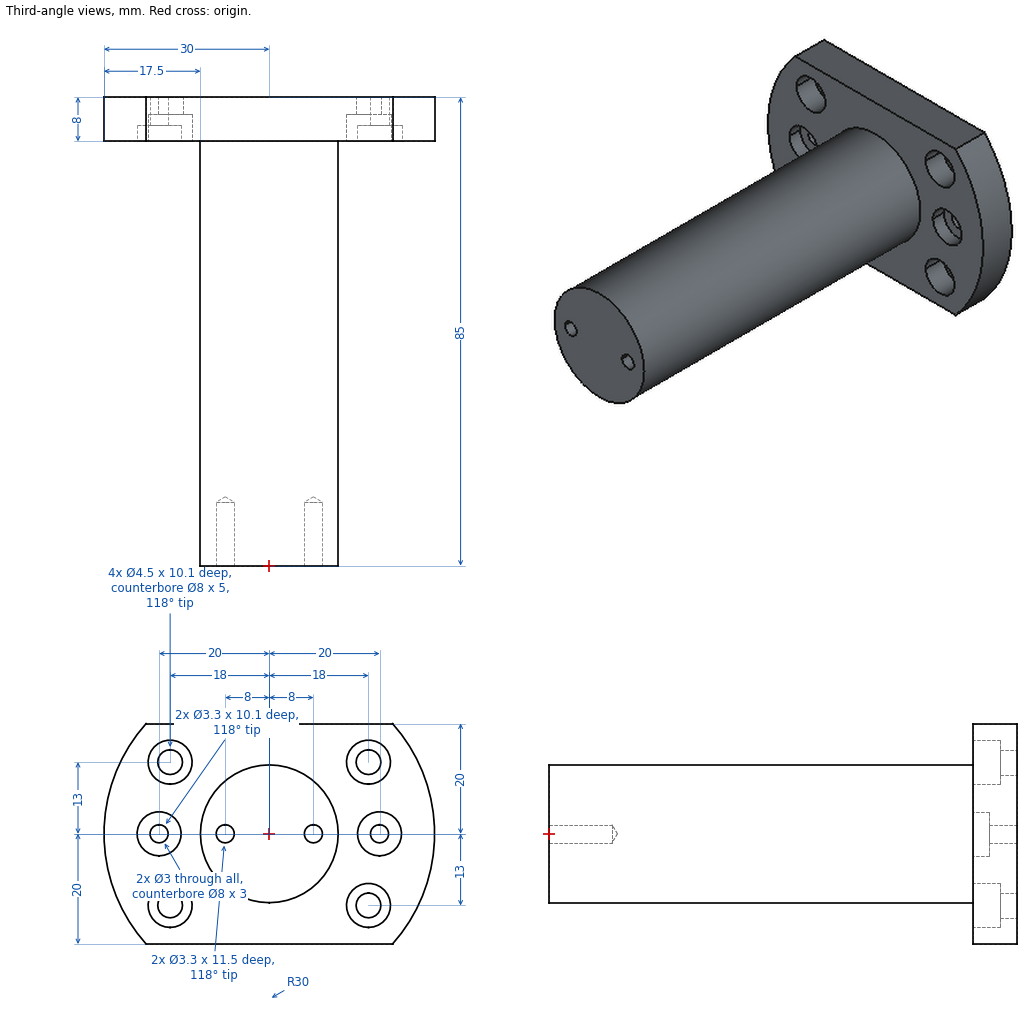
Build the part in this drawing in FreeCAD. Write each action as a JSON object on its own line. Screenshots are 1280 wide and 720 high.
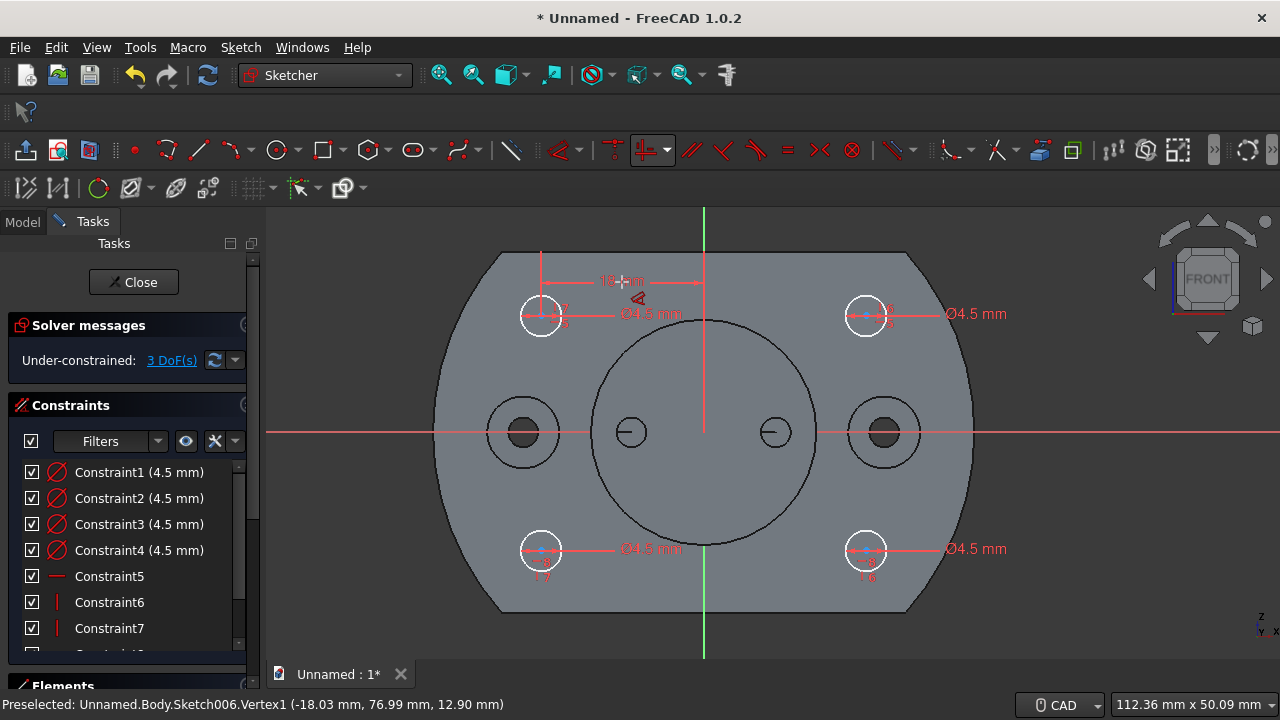
{"action": "left_click", "coordinate": [541, 316]}
{"action": "left_click", "coordinate": [507, 374]}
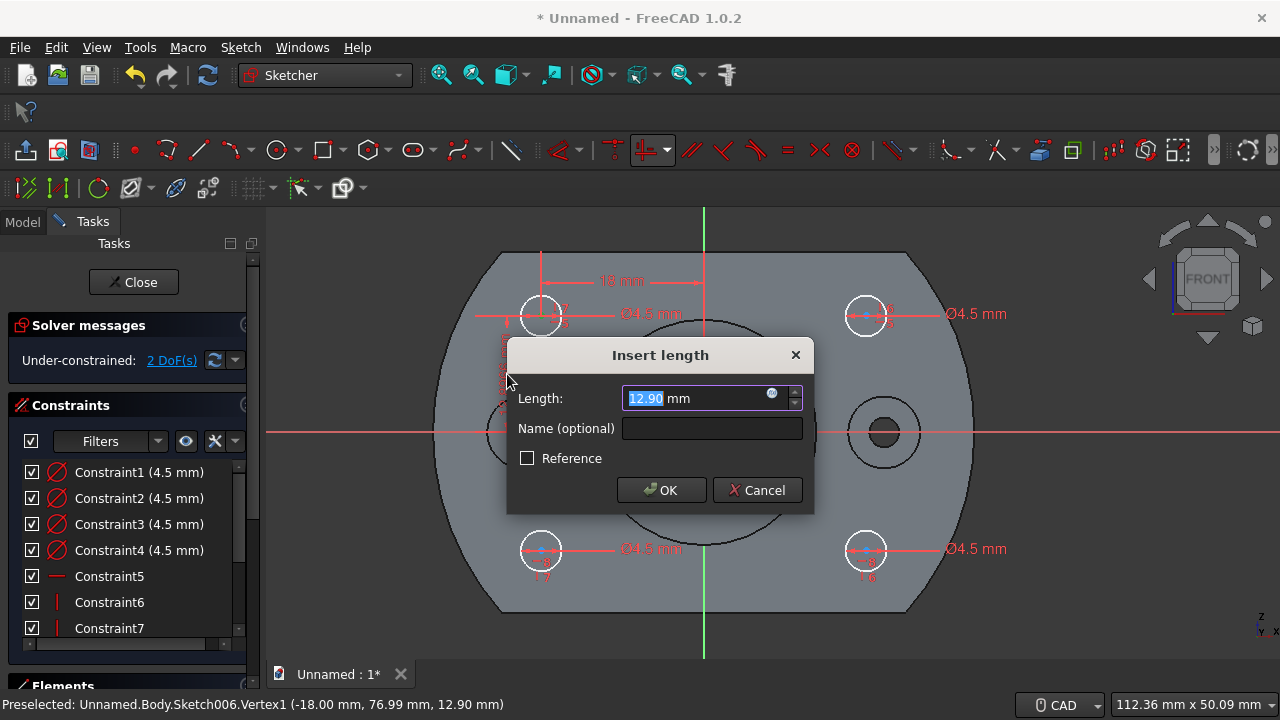
{"action": "type", "text": "13"}
{"action": "key", "text": "Return"}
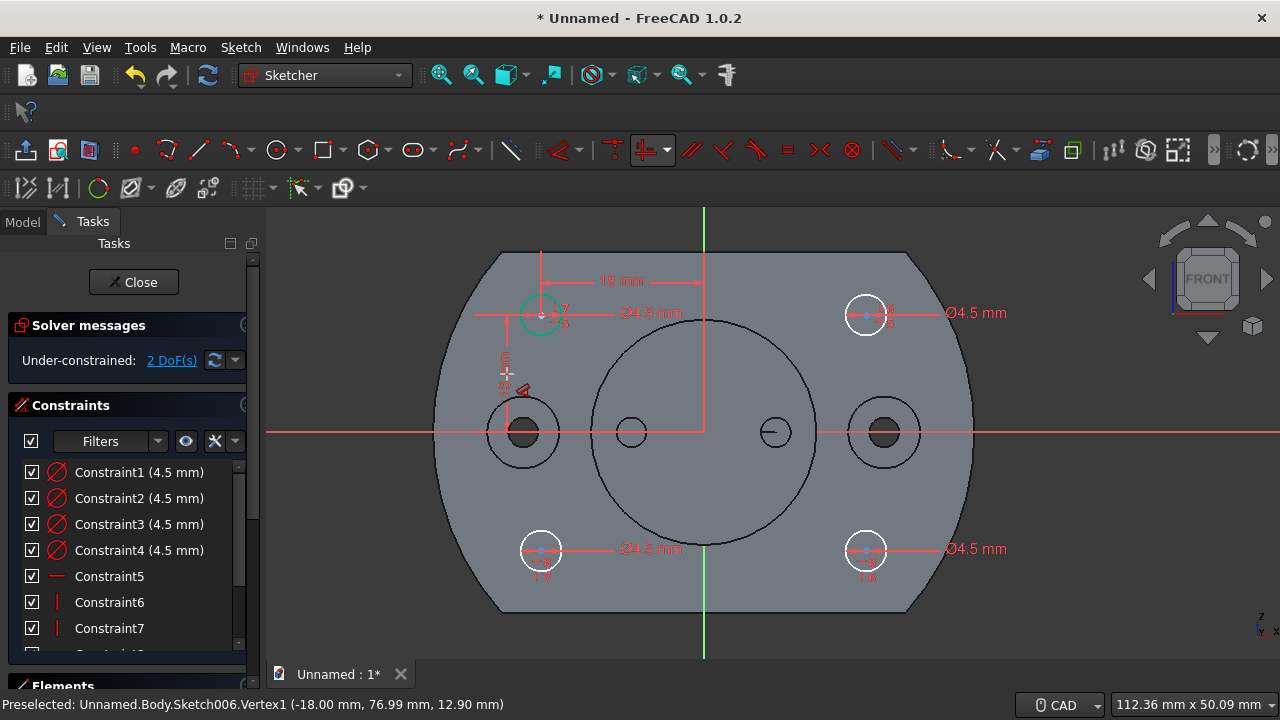
{"action": "left_click", "coordinate": [866, 315]}
{"action": "left_click", "coordinate": [785, 281]}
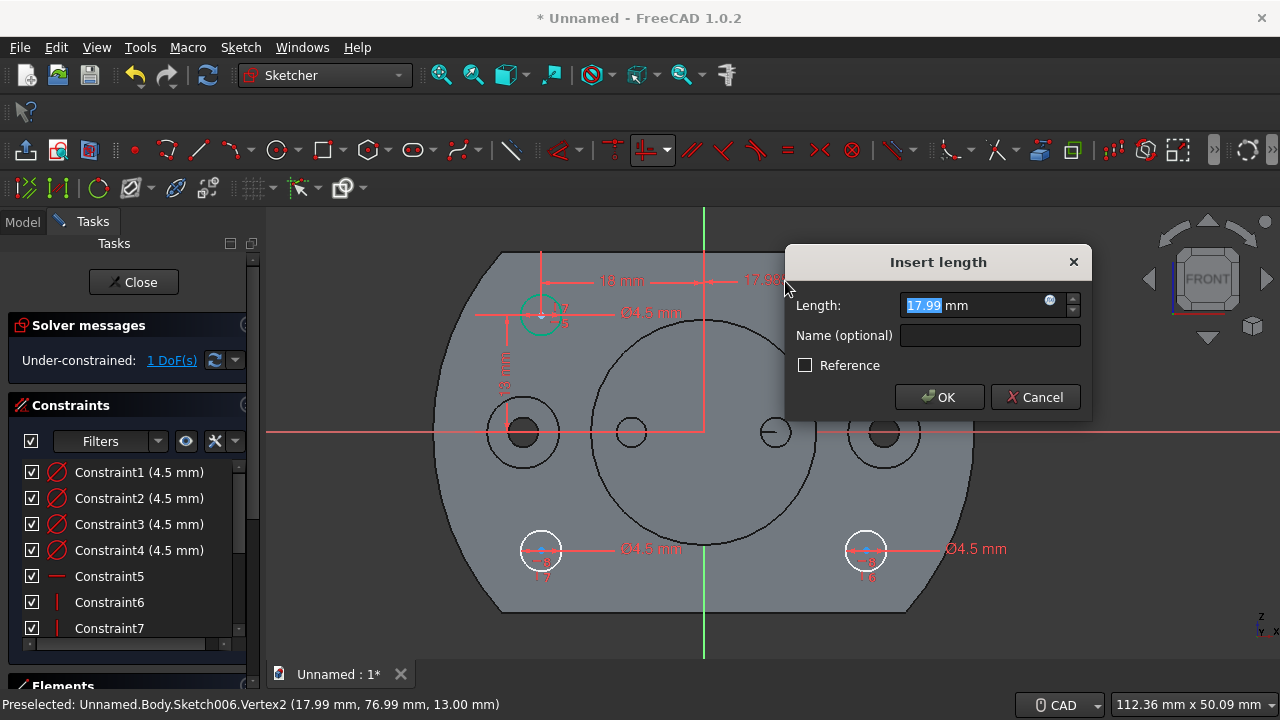
{"action": "type", "text": "18"}
{"action": "key", "text": "Return"}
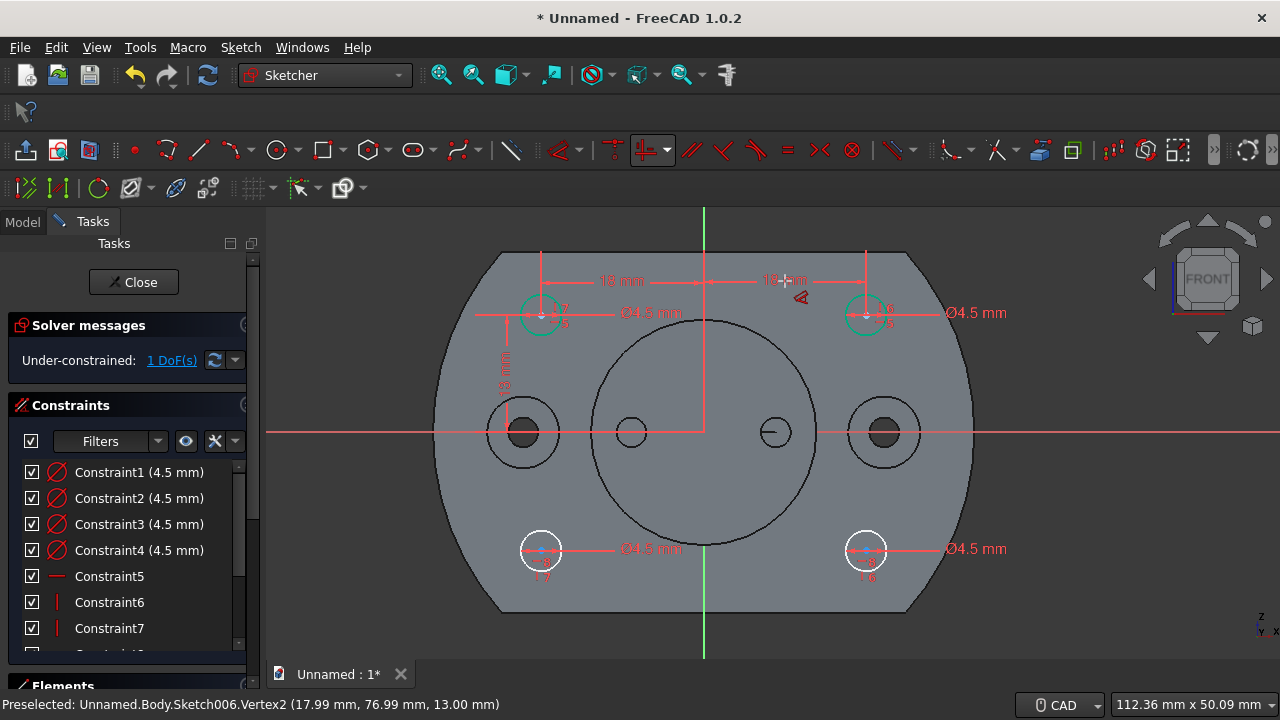
{"action": "left_click", "coordinate": [866, 551]}
{"action": "left_click", "coordinate": [900, 492]}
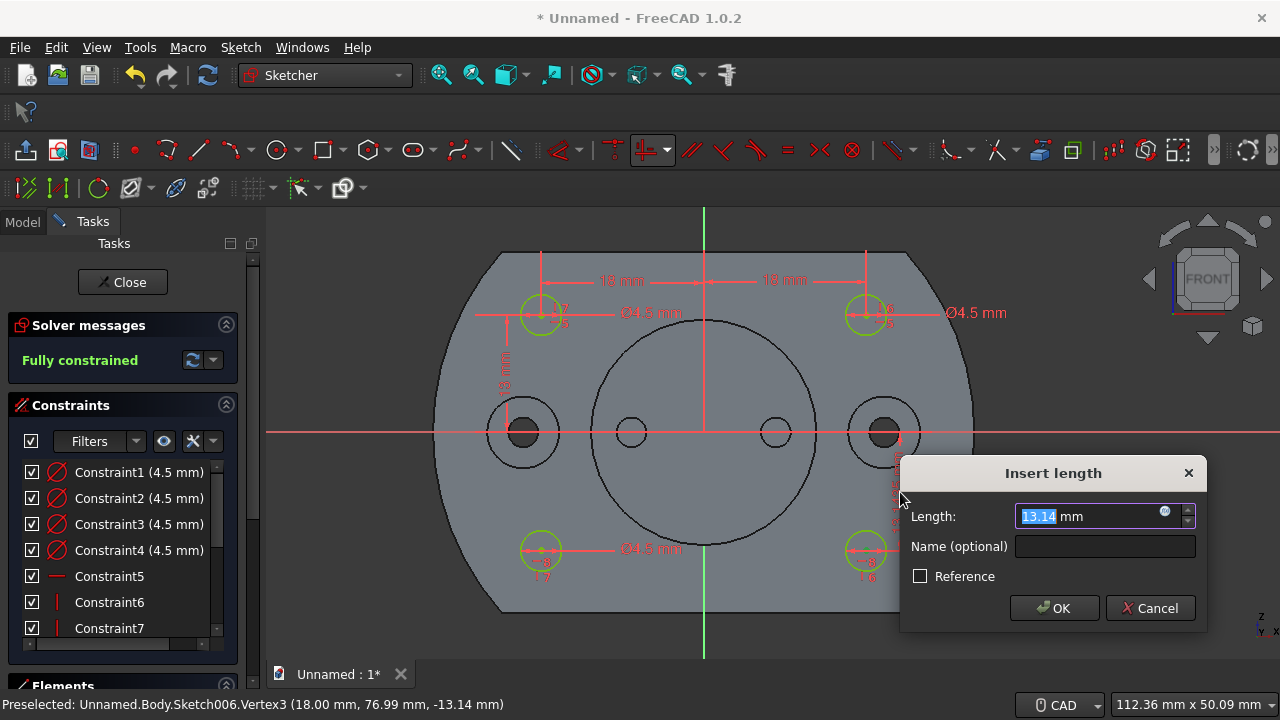
{"action": "type", "text": "13"}
{"action": "key", "text": "Return"}
{"action": "key", "text": "Escape"}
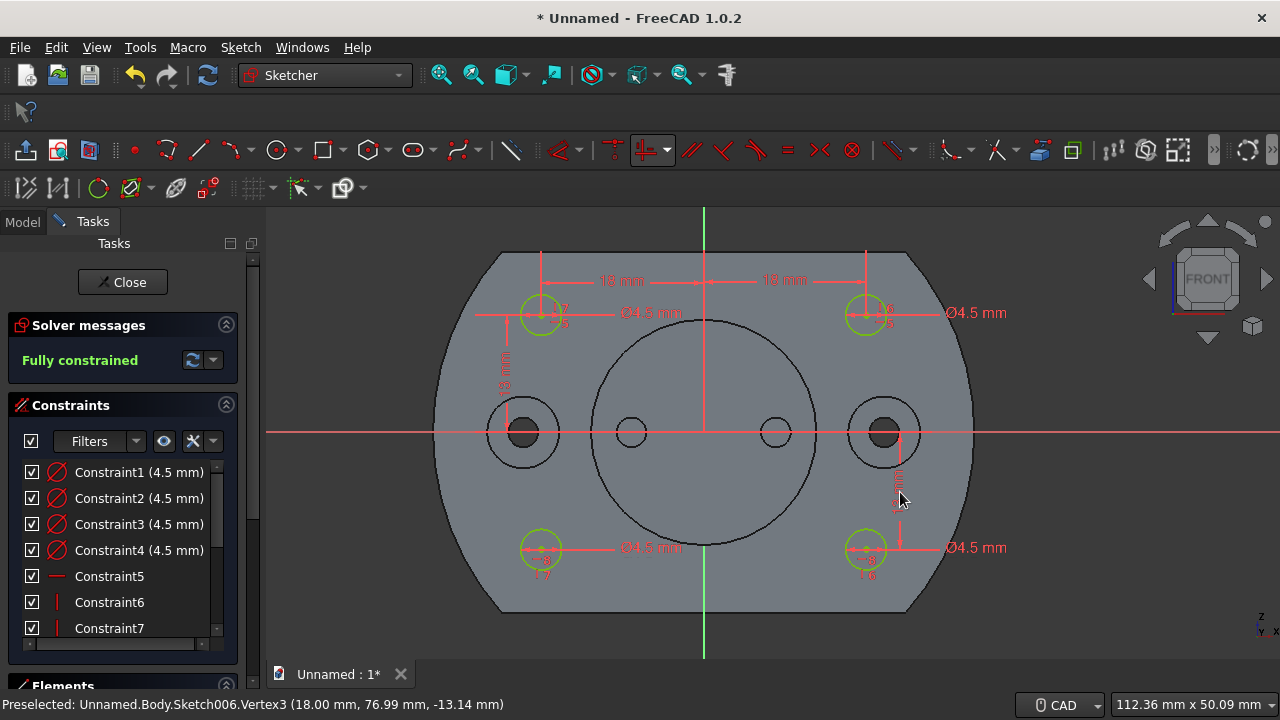
{"action": "left_click", "coordinate": [123, 282]}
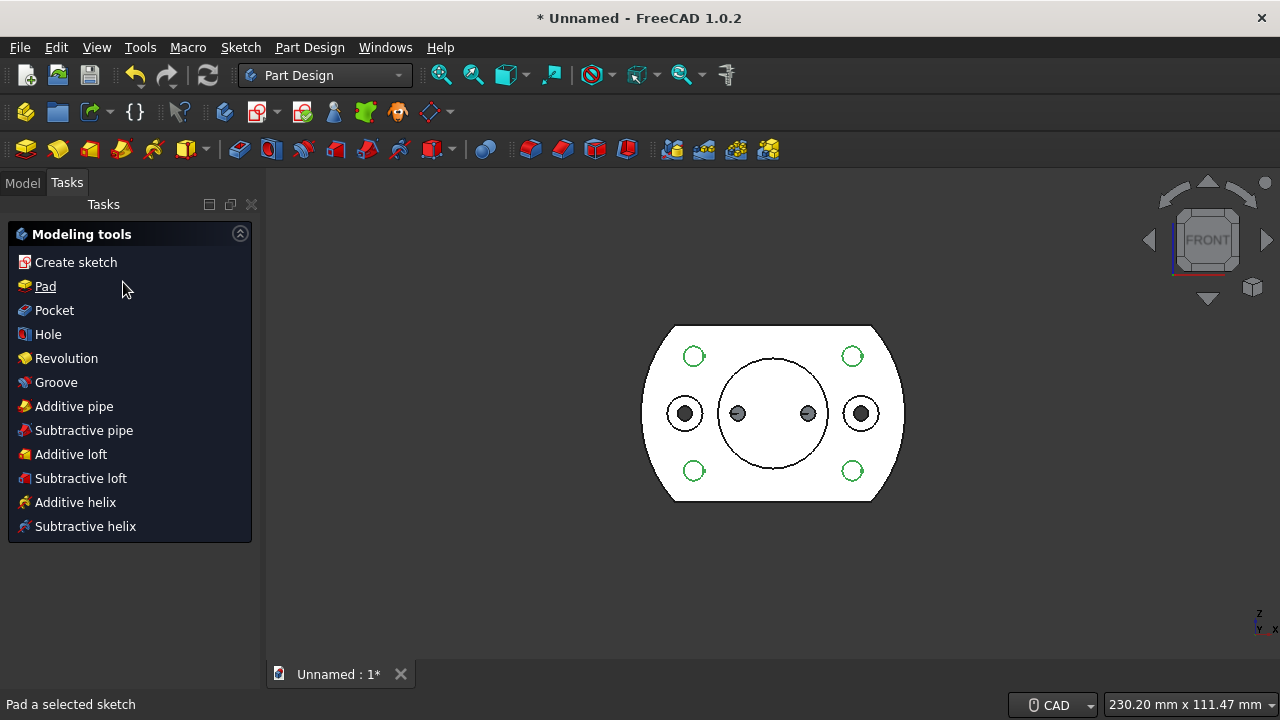
{"action": "left_click", "coordinate": [272, 150]}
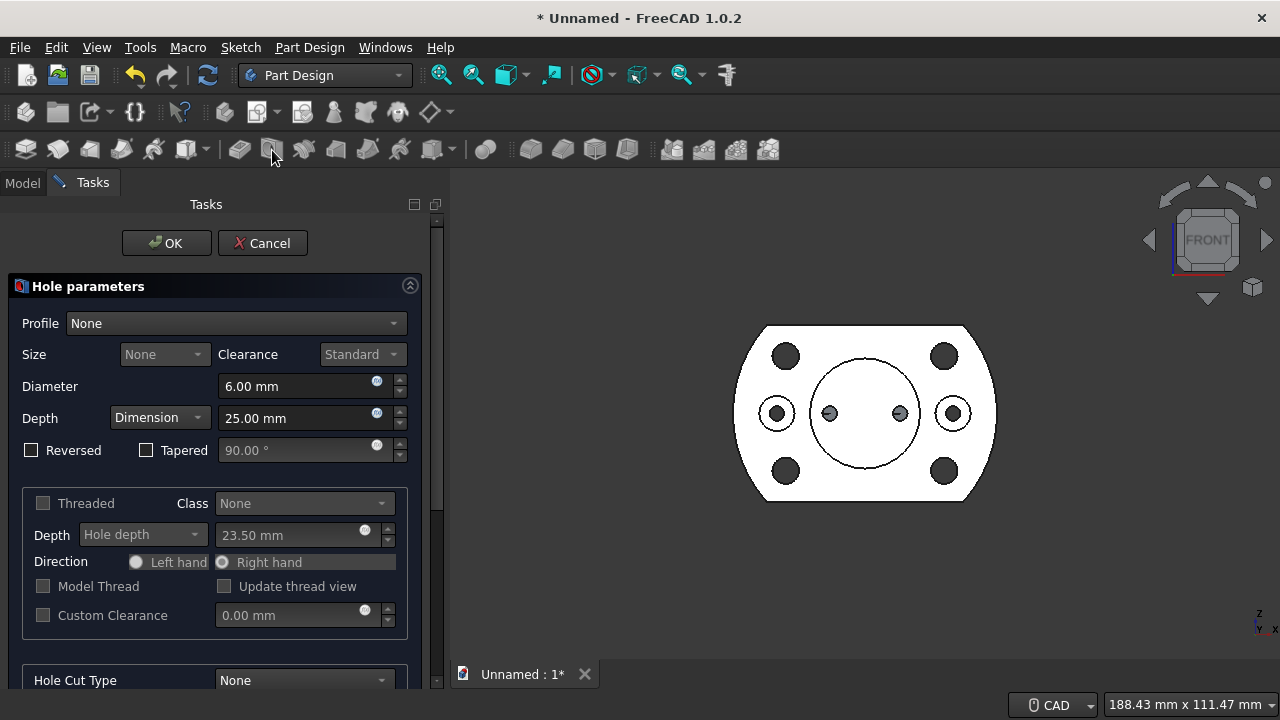
{"action": "triple_click", "coordinate": [305, 386]}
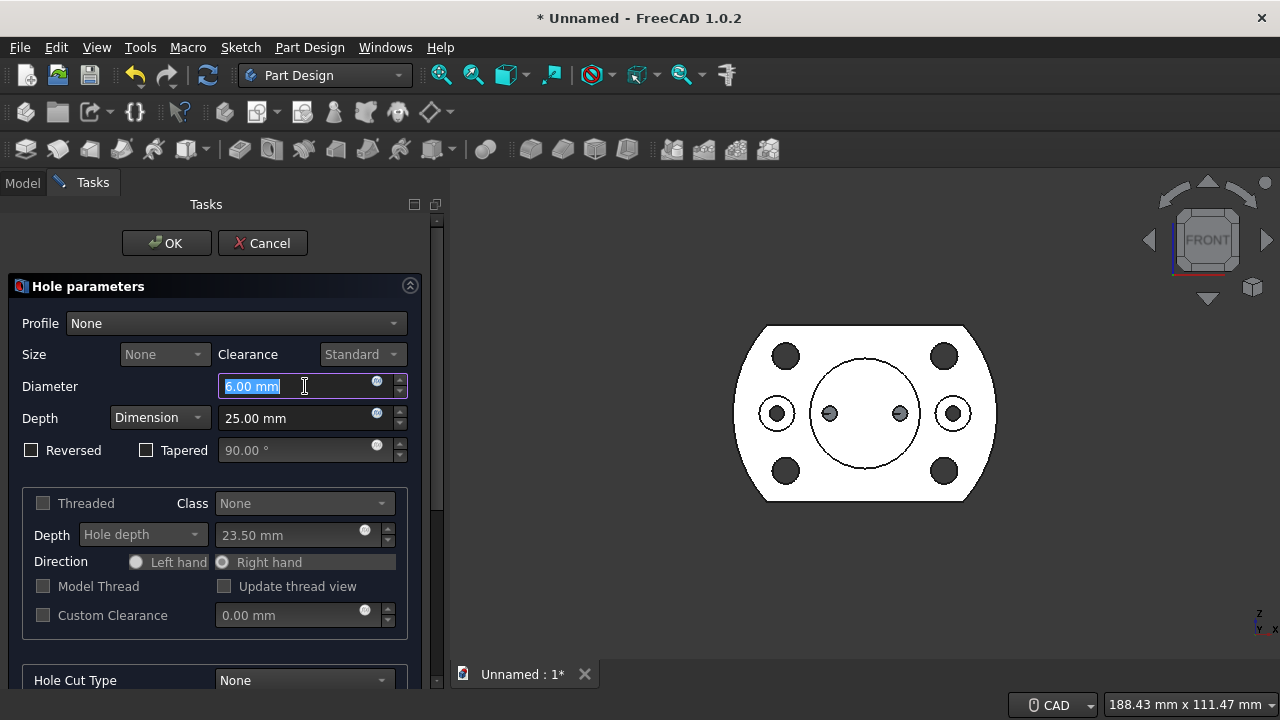
{"action": "type", "text": "4.5"}
{"action": "key", "text": "Tab"}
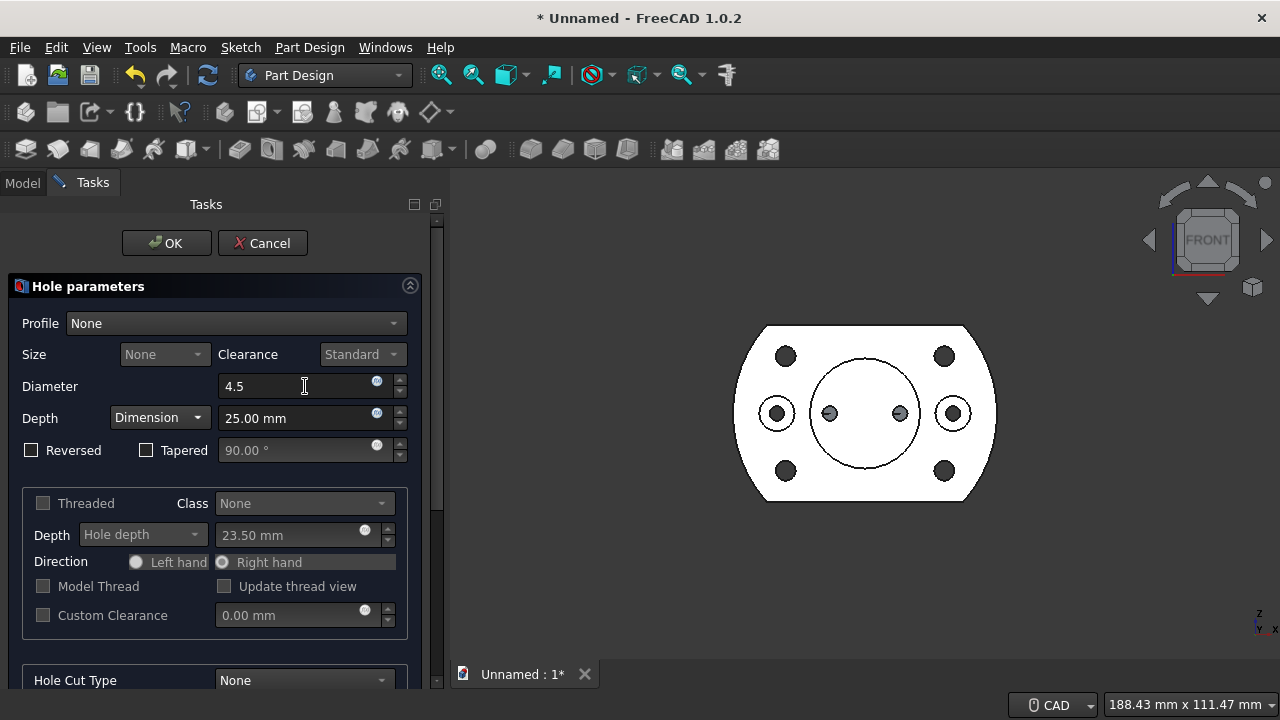
{"action": "triple_click", "coordinate": [305, 418]}